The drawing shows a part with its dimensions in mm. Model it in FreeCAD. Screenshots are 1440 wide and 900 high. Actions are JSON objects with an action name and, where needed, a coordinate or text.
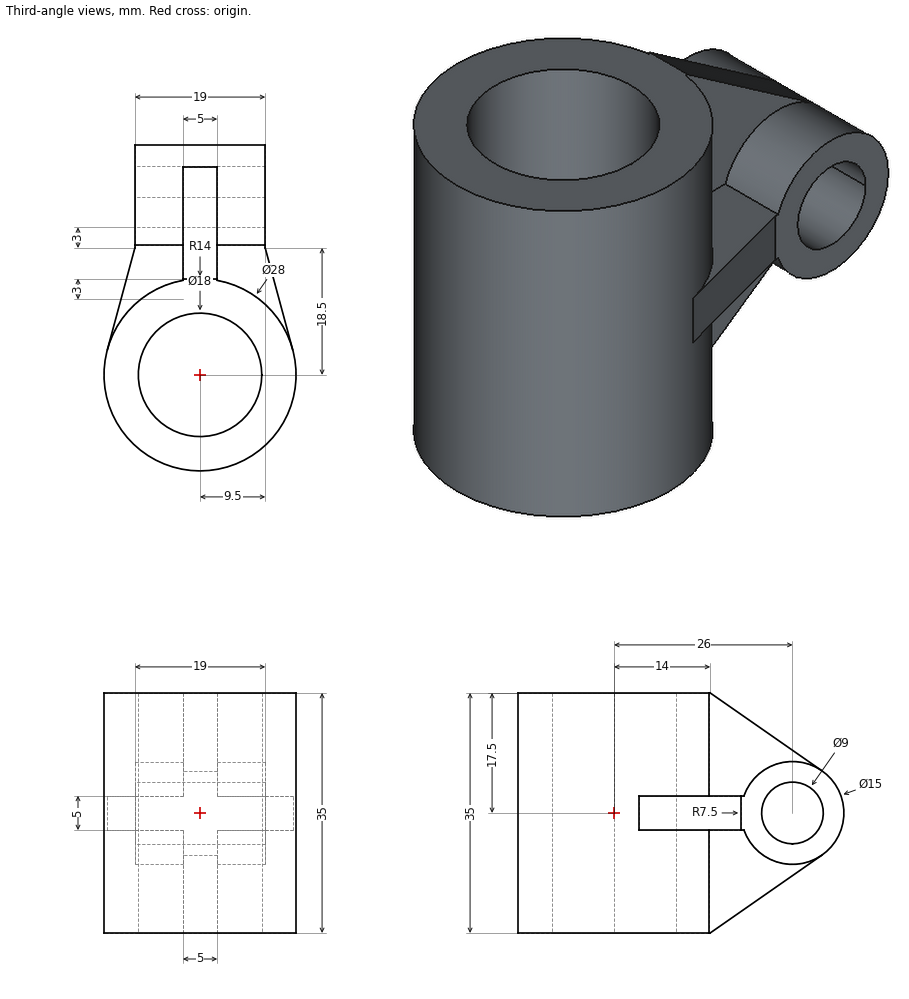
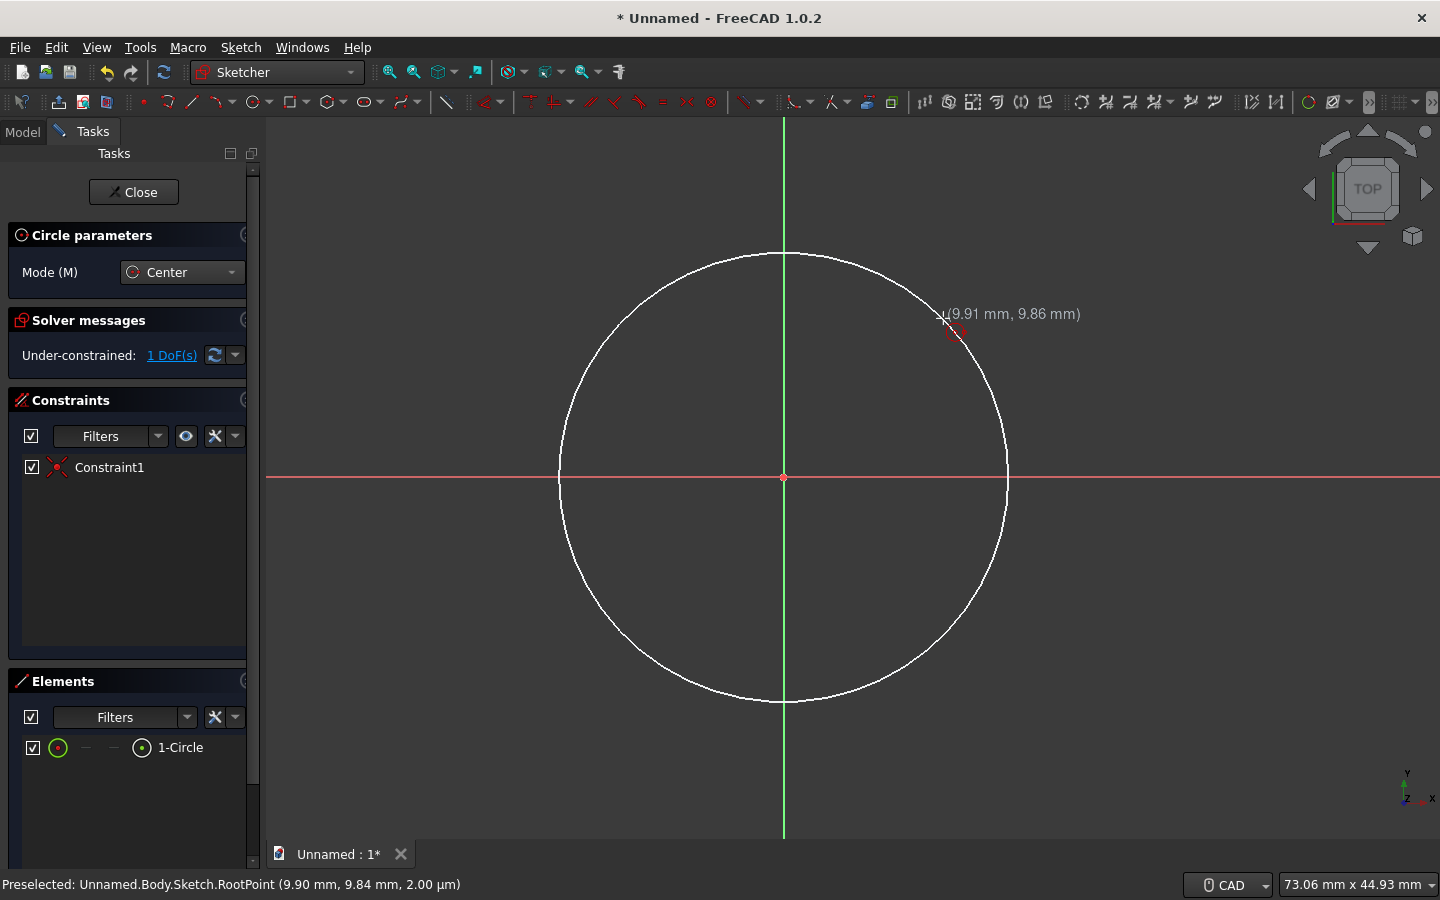
{"action": "left_click", "coordinate": [784, 477]}
{"action": "left_click", "coordinate": [886, 375]}
{"action": "key", "text": "Escape"}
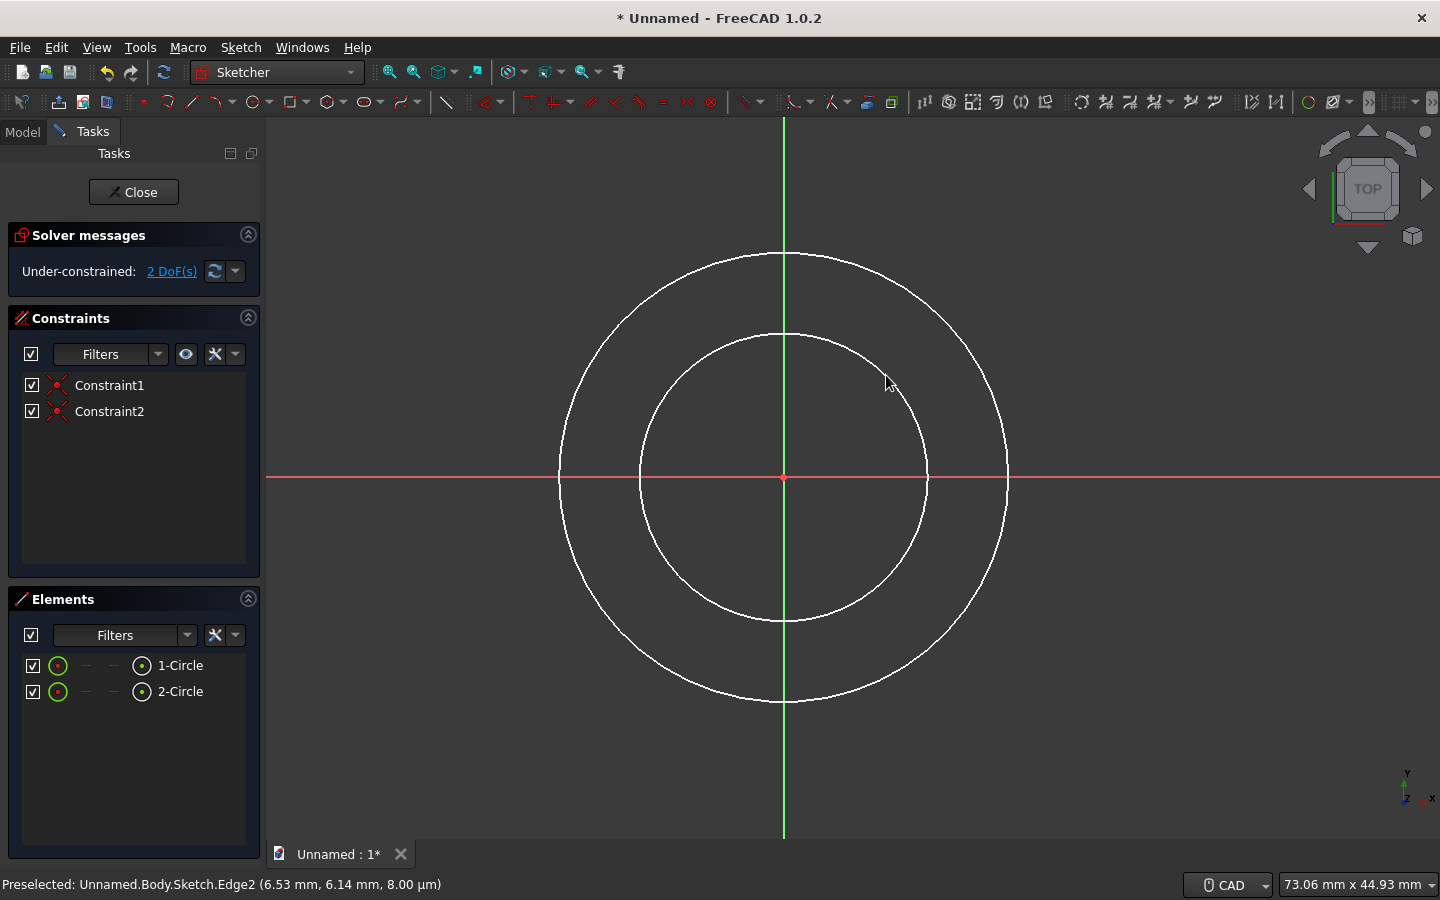
{"action": "key", "text": "d"}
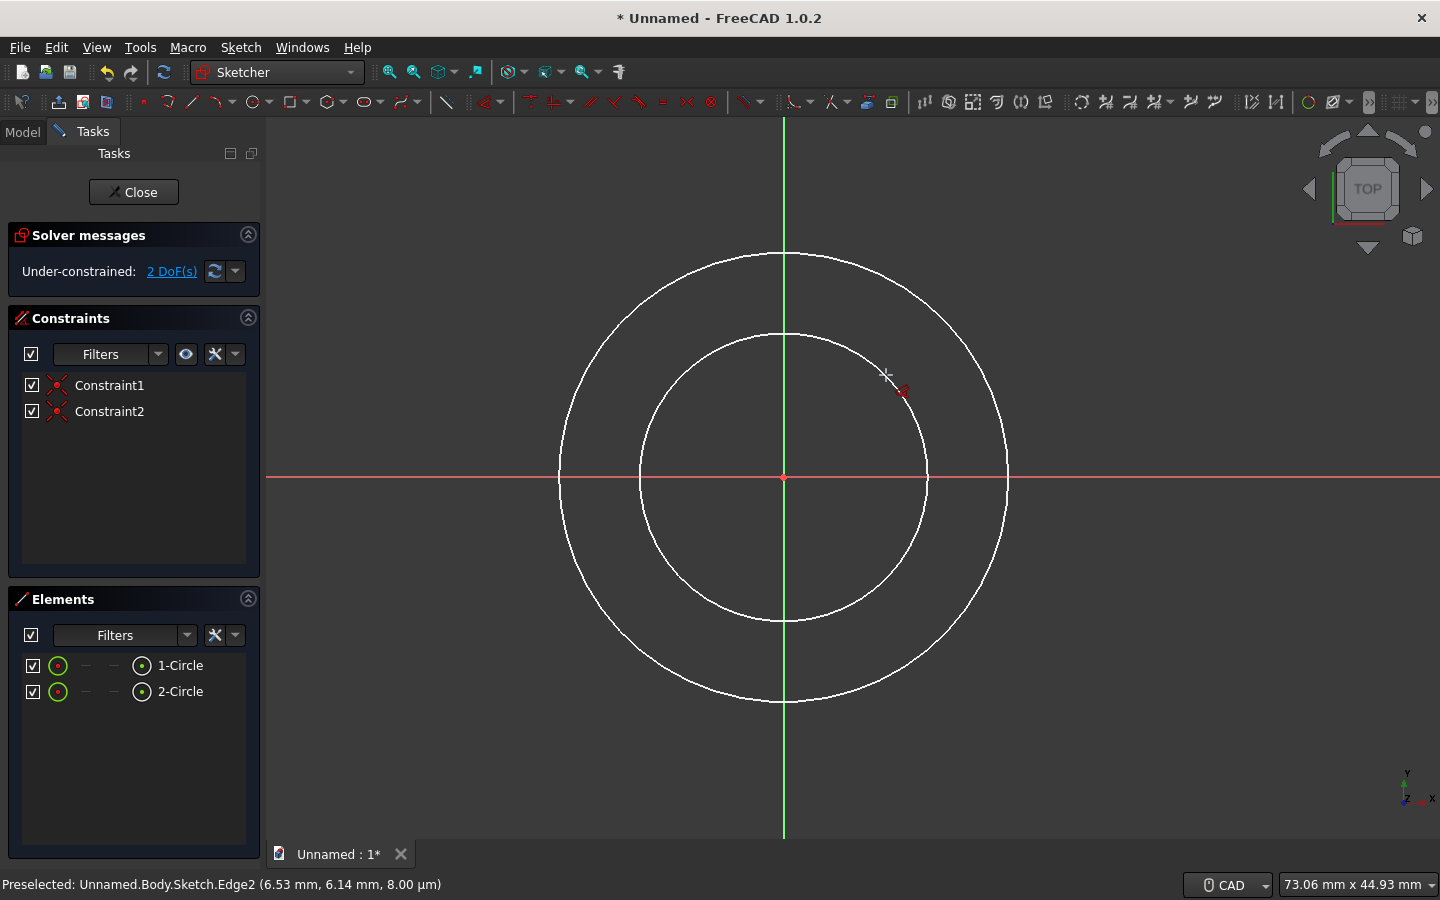
{"action": "left_click", "coordinate": [942, 318]}
{"action": "left_click", "coordinate": [965, 295]}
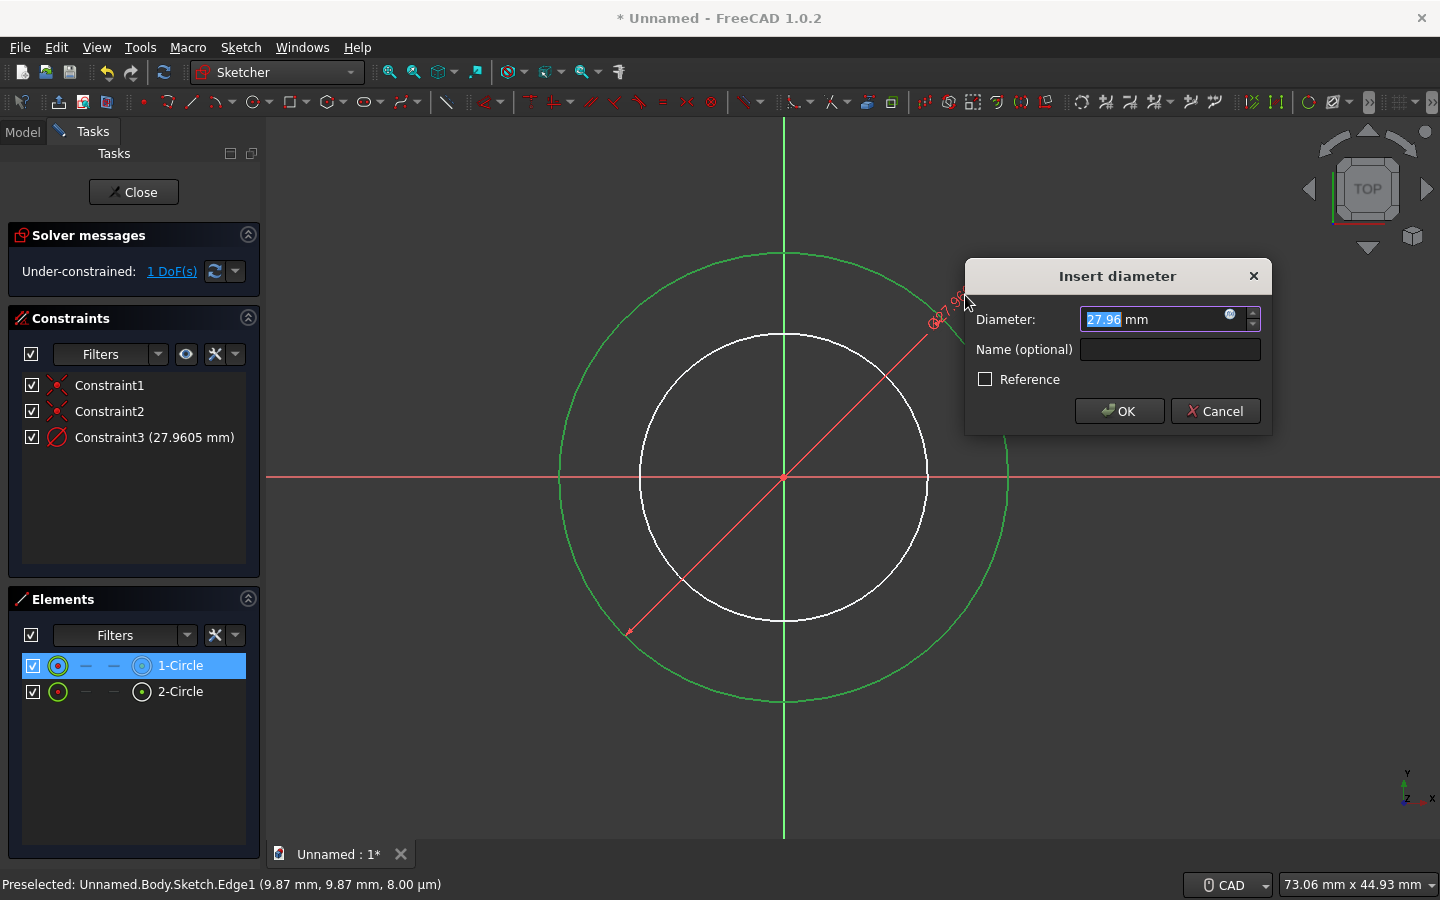
{"action": "type", "text": "28"}
{"action": "key", "text": "Return"}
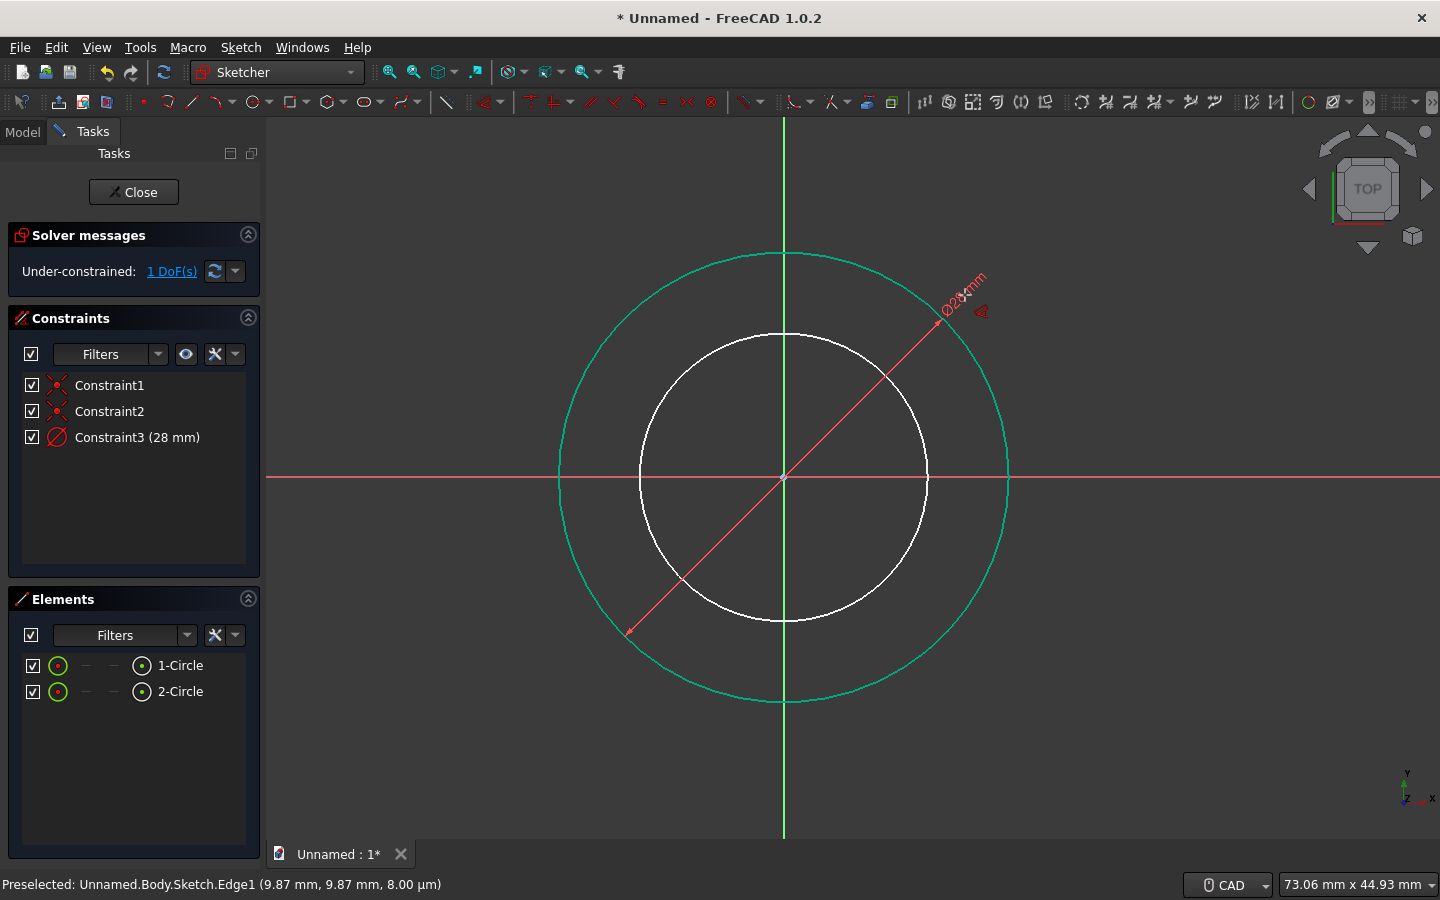
{"action": "left_click", "coordinate": [885, 375]}
{"action": "left_click", "coordinate": [908, 352]}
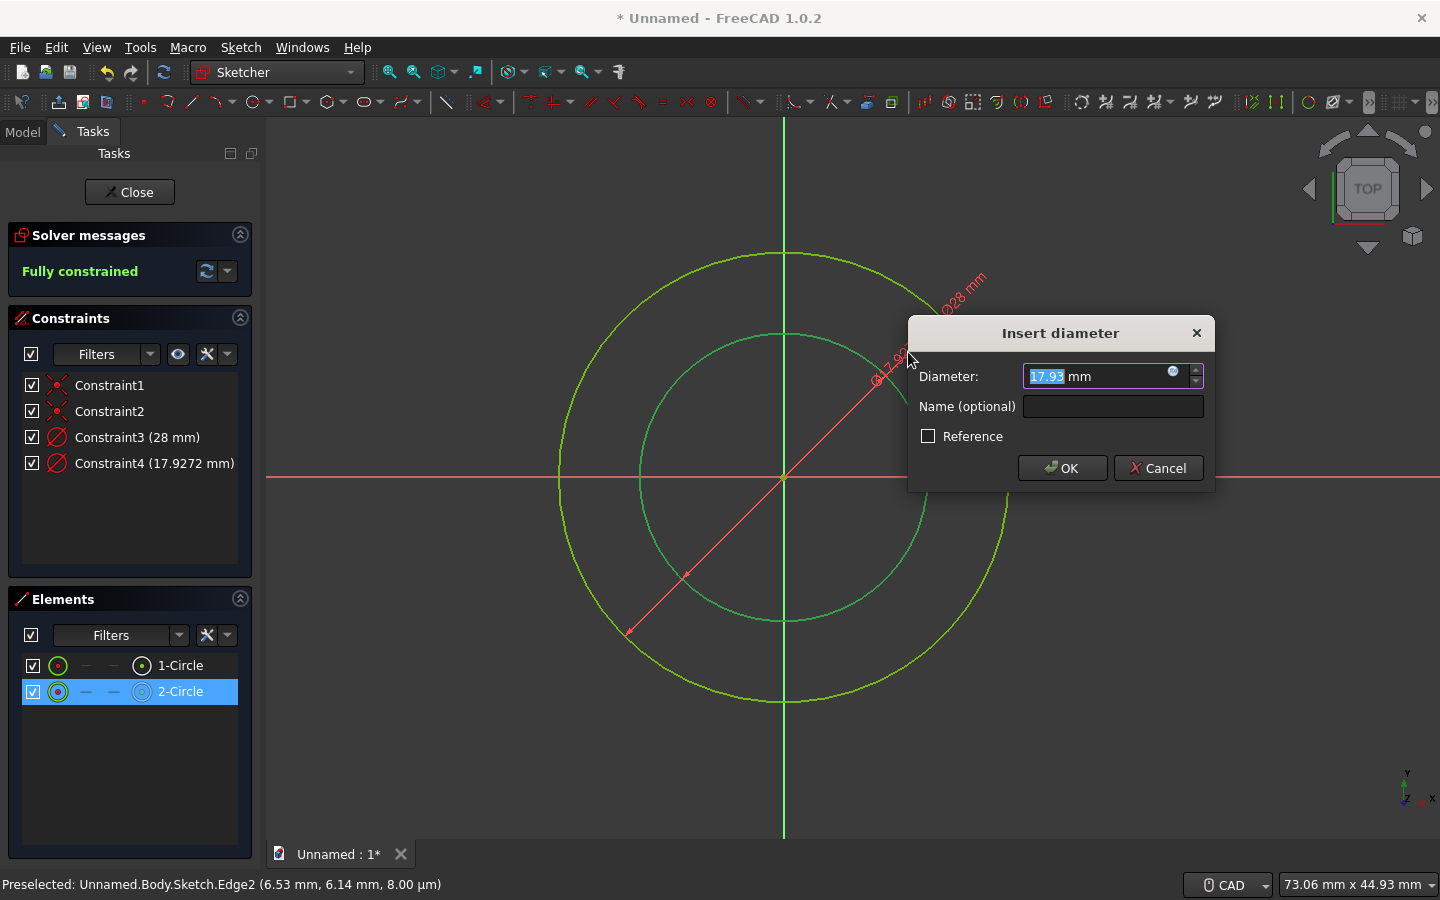
{"action": "type", "text": "18"}
{"action": "key", "text": "Return"}
{"action": "key", "text": "Escape"}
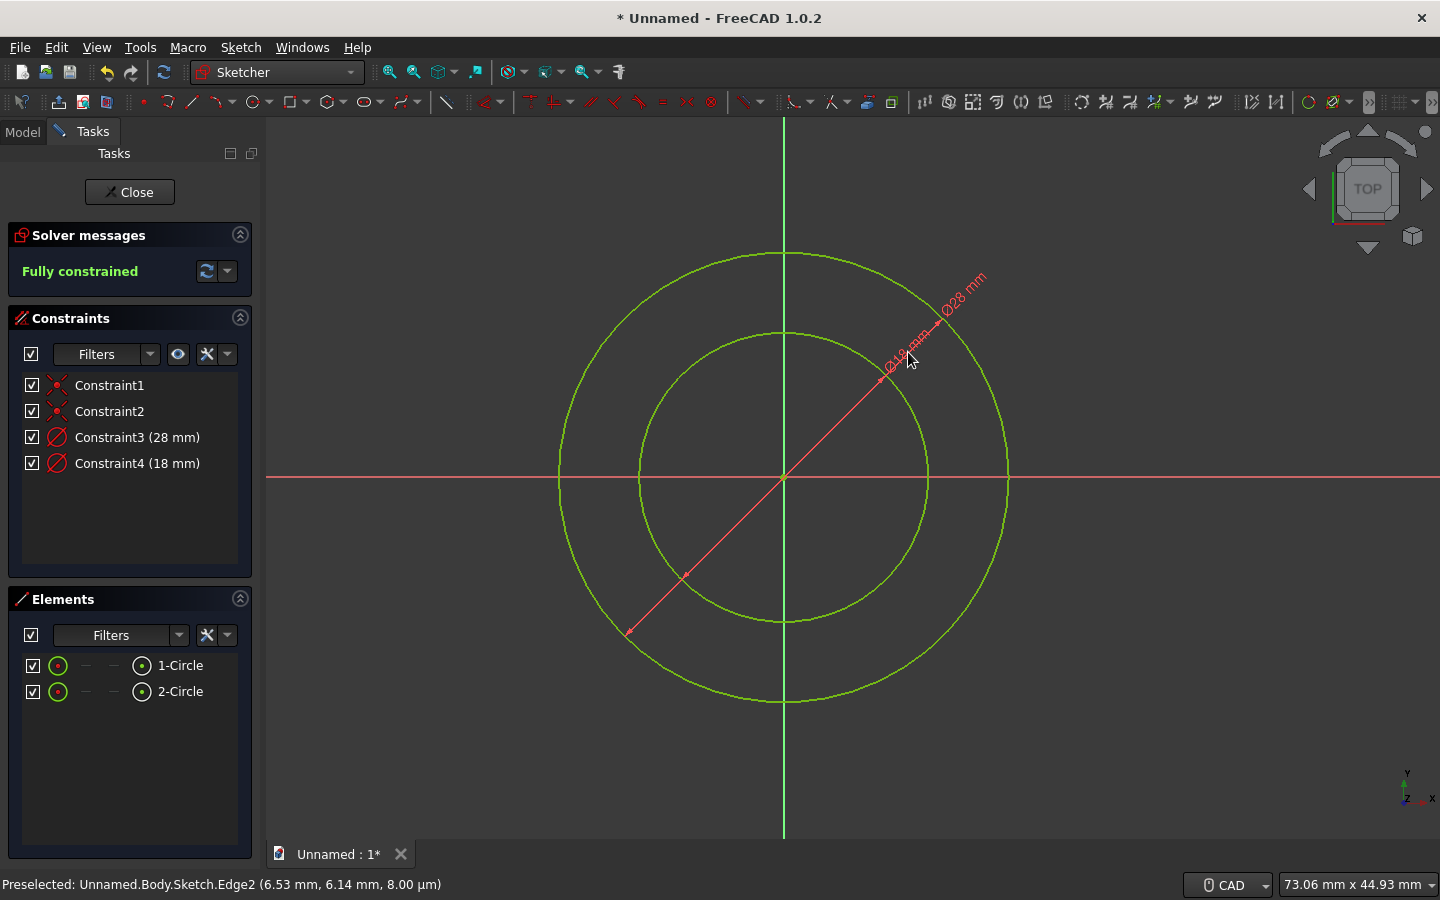
{"action": "left_click", "coordinate": [130, 192]}